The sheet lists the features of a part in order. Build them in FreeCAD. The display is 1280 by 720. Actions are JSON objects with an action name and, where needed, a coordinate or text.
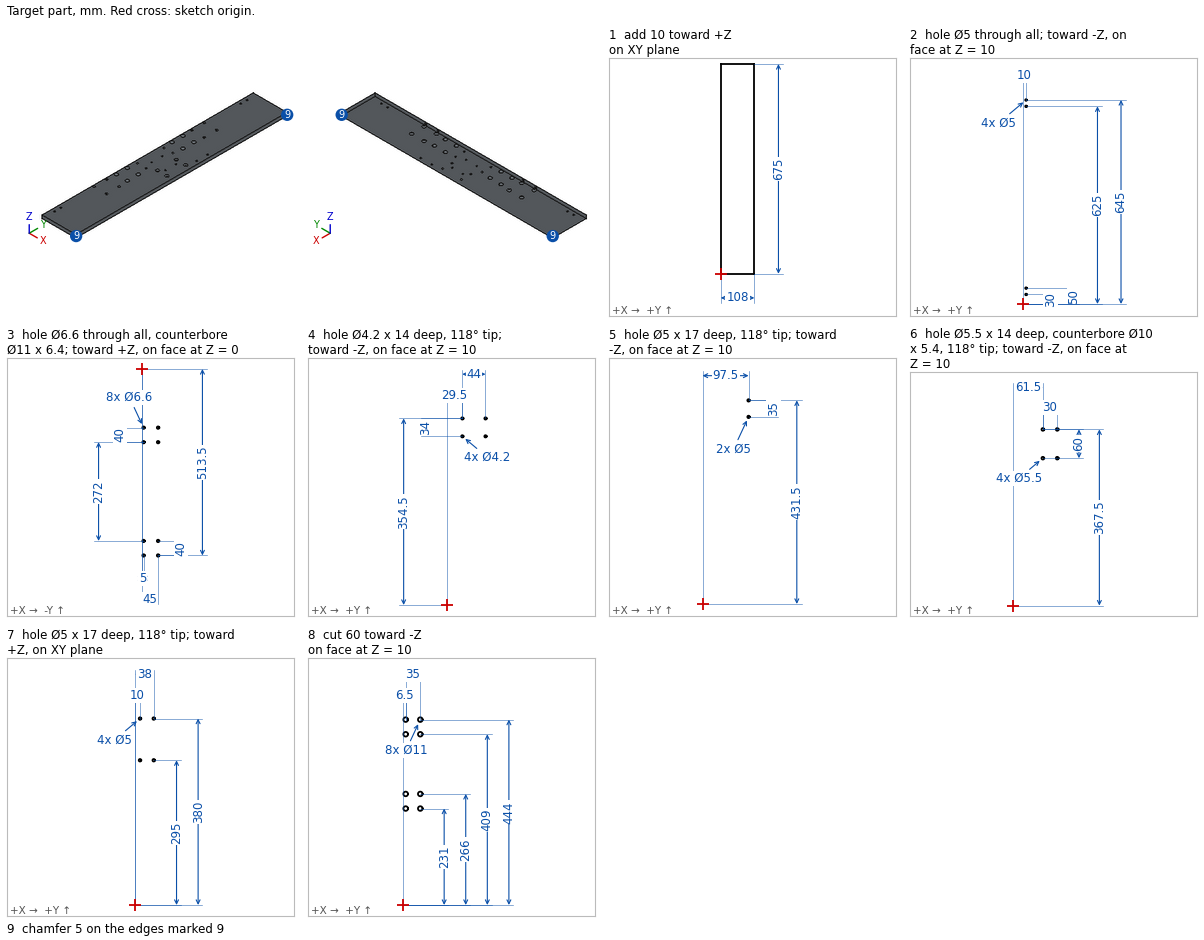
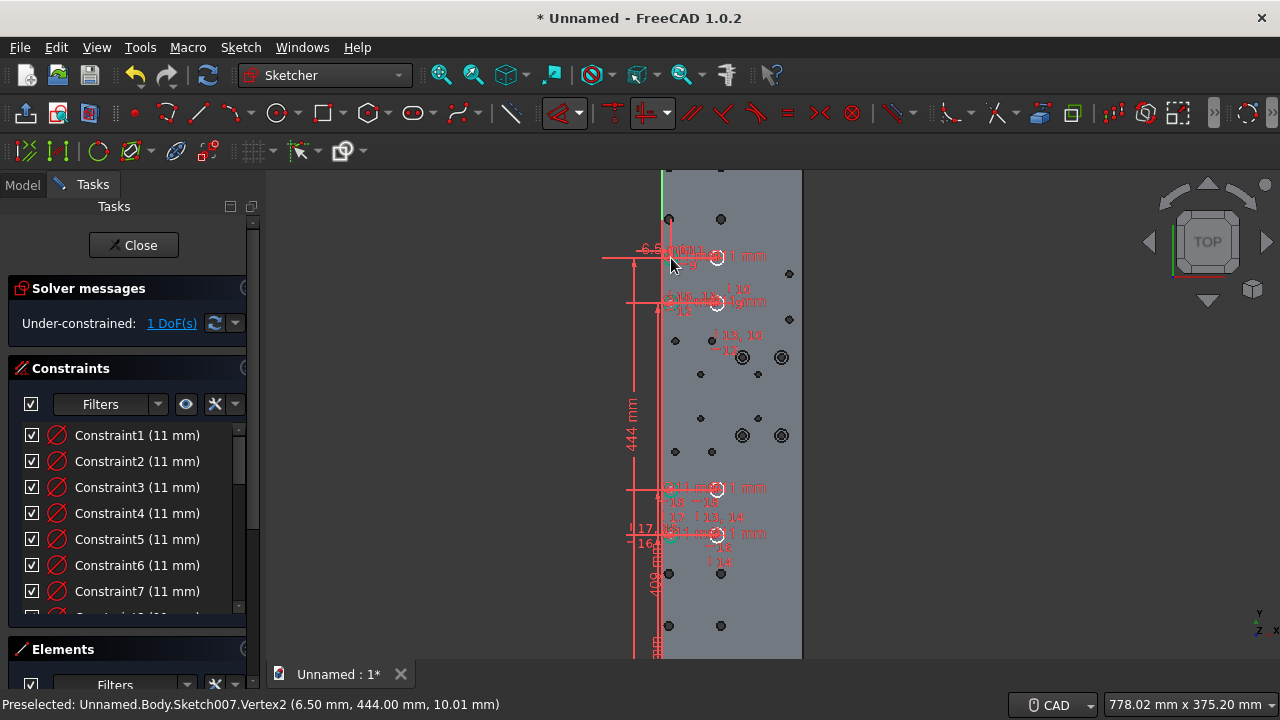
{"action": "key", "text": "l"}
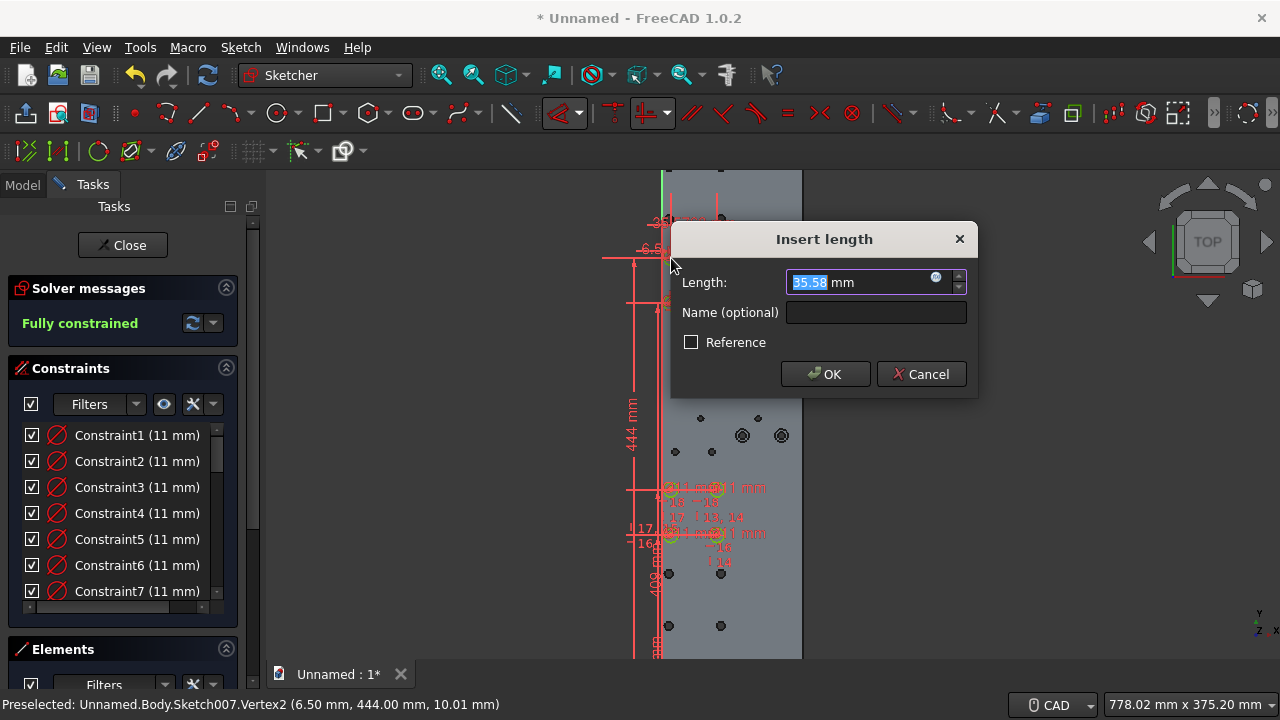
{"action": "type", "text": "35"}
{"action": "key", "text": "Return"}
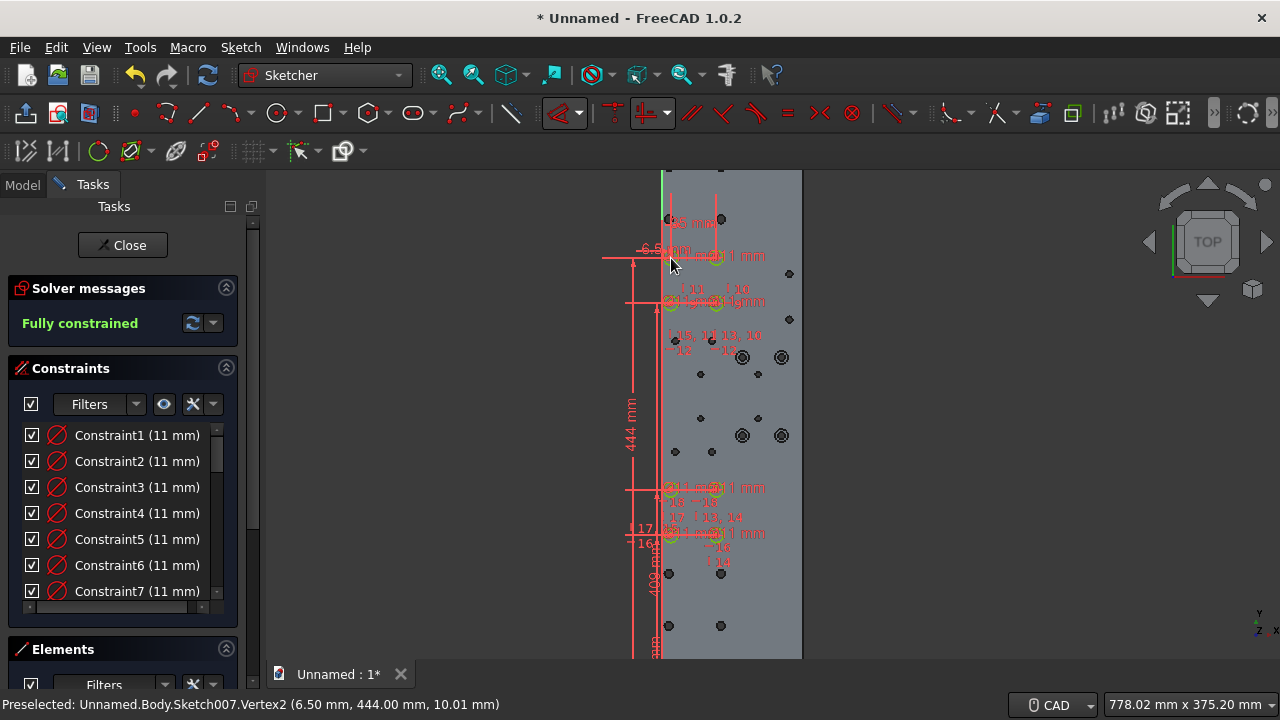
{"action": "left_click", "coordinate": [123, 245]}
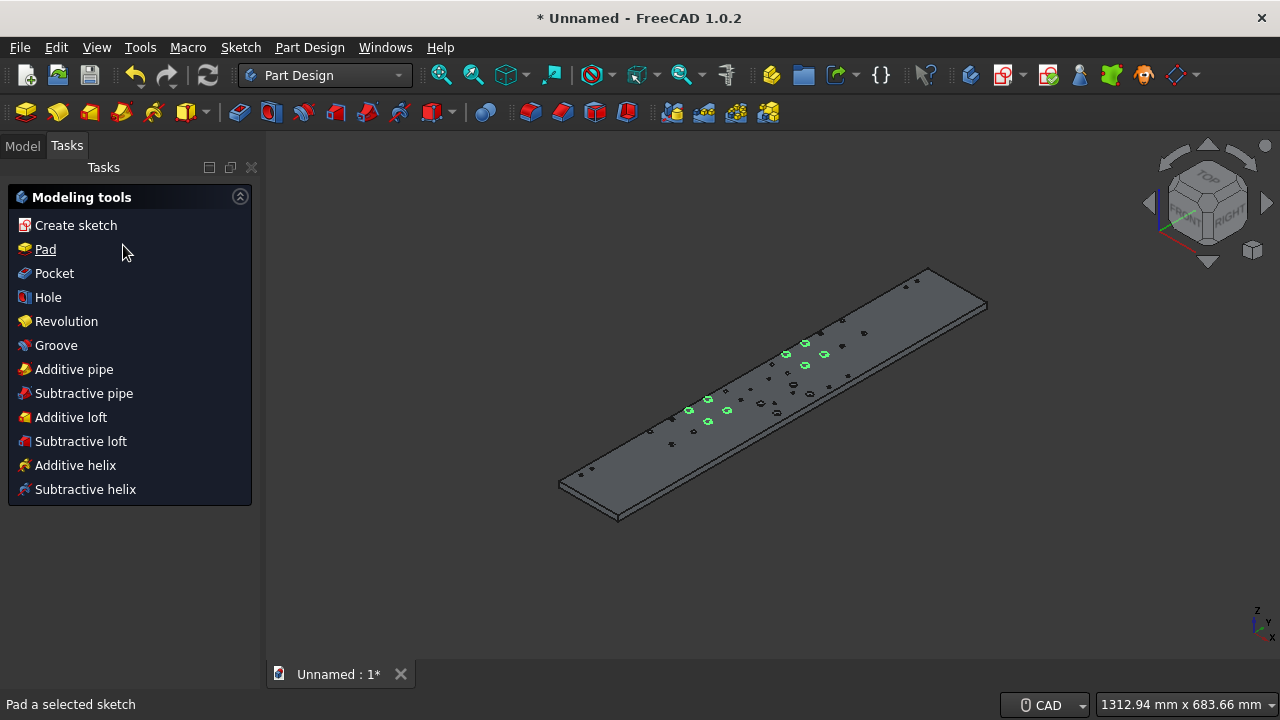
{"action": "left_click", "coordinate": [240, 112]}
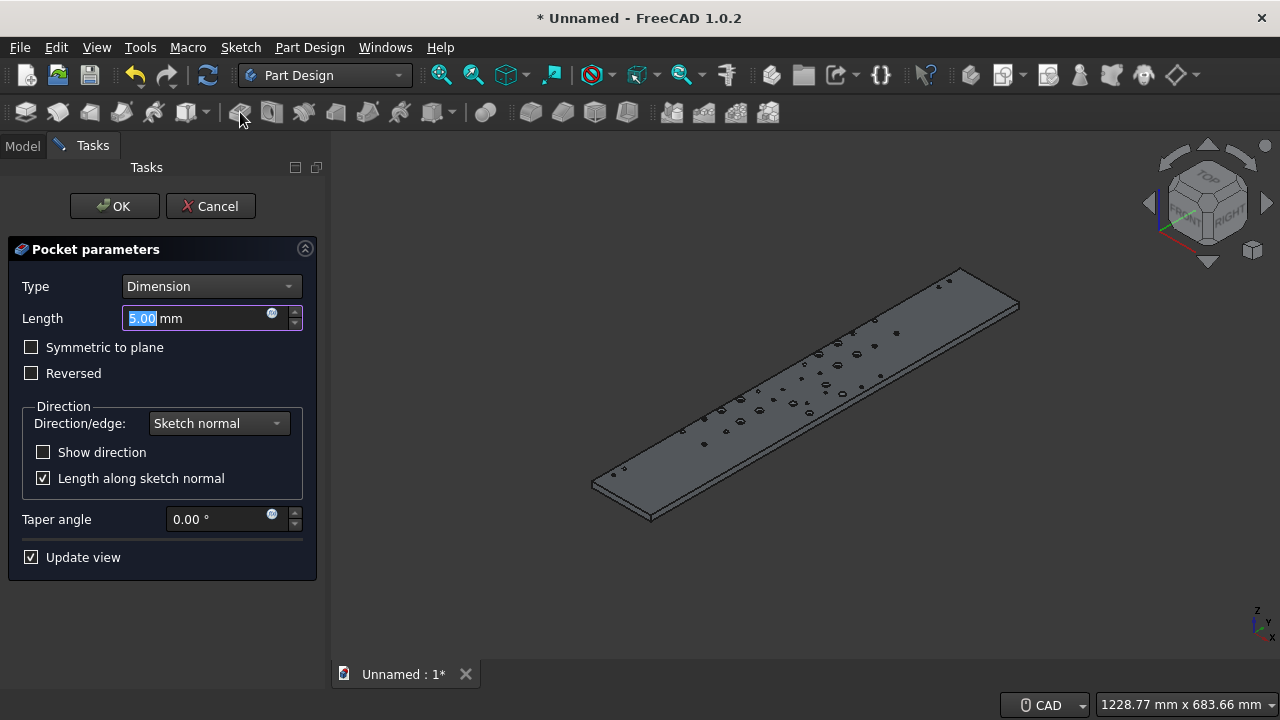
{"action": "type", "text": "60"}
{"action": "key", "text": "Tab"}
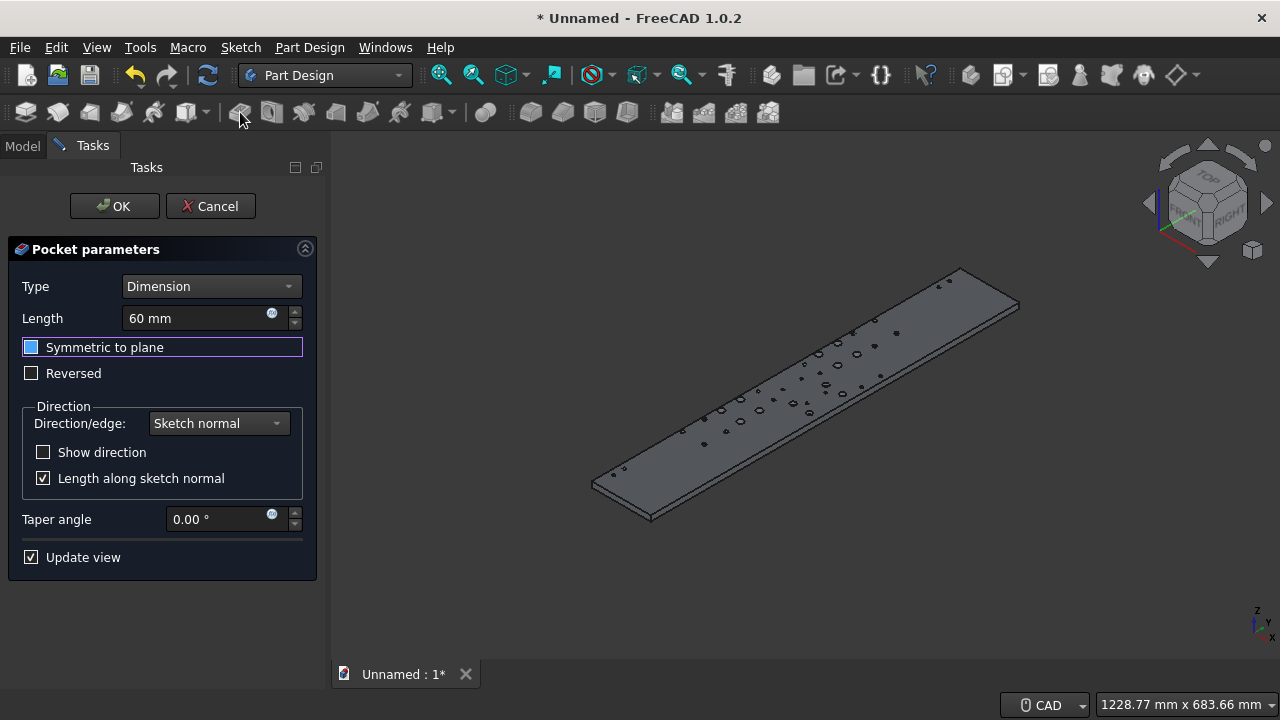
{"action": "left_click", "coordinate": [115, 206]}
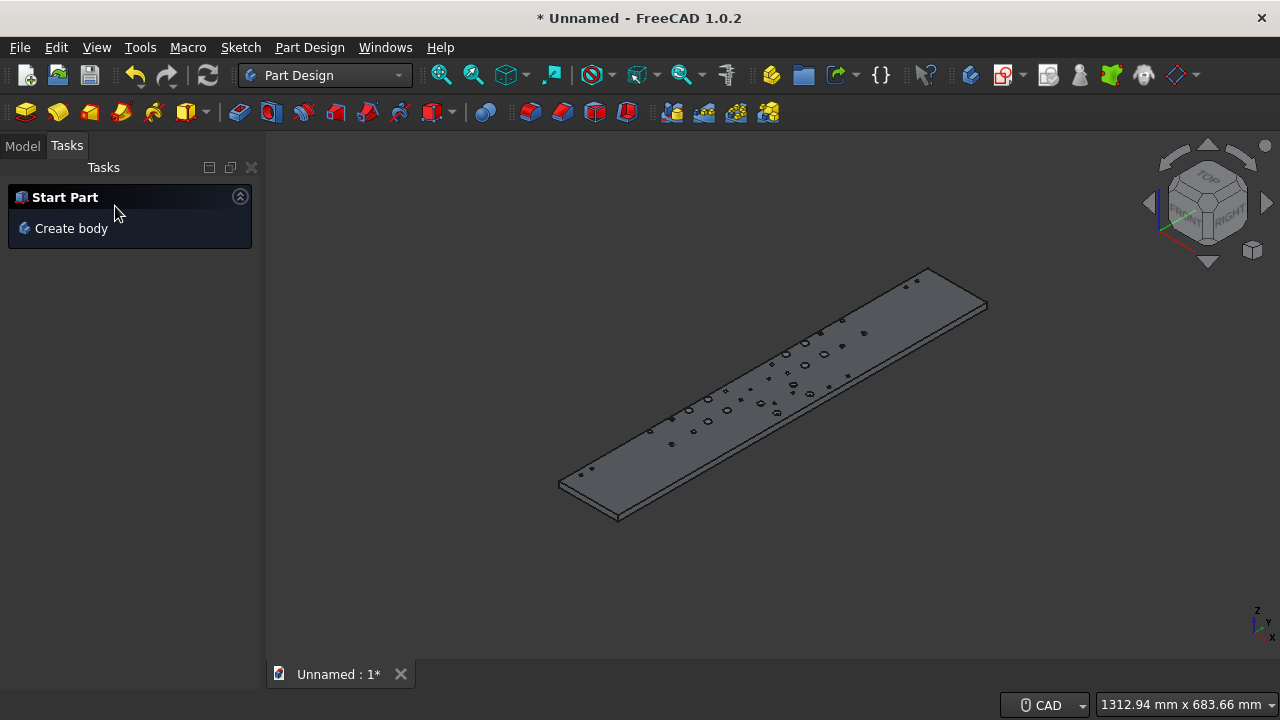
{"action": "scroll", "coordinate": [618, 517], "scroll_direction": "up", "scroll_amount": 9}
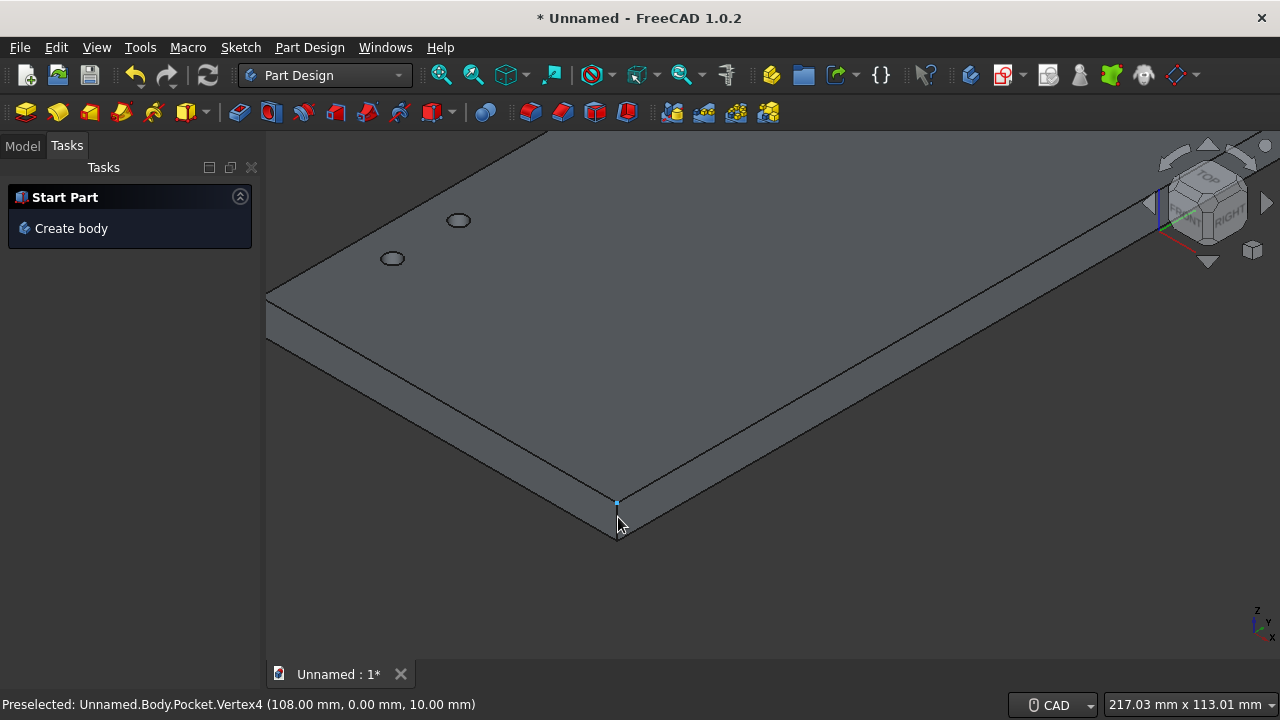
{"action": "left_click", "coordinate": [617, 521]}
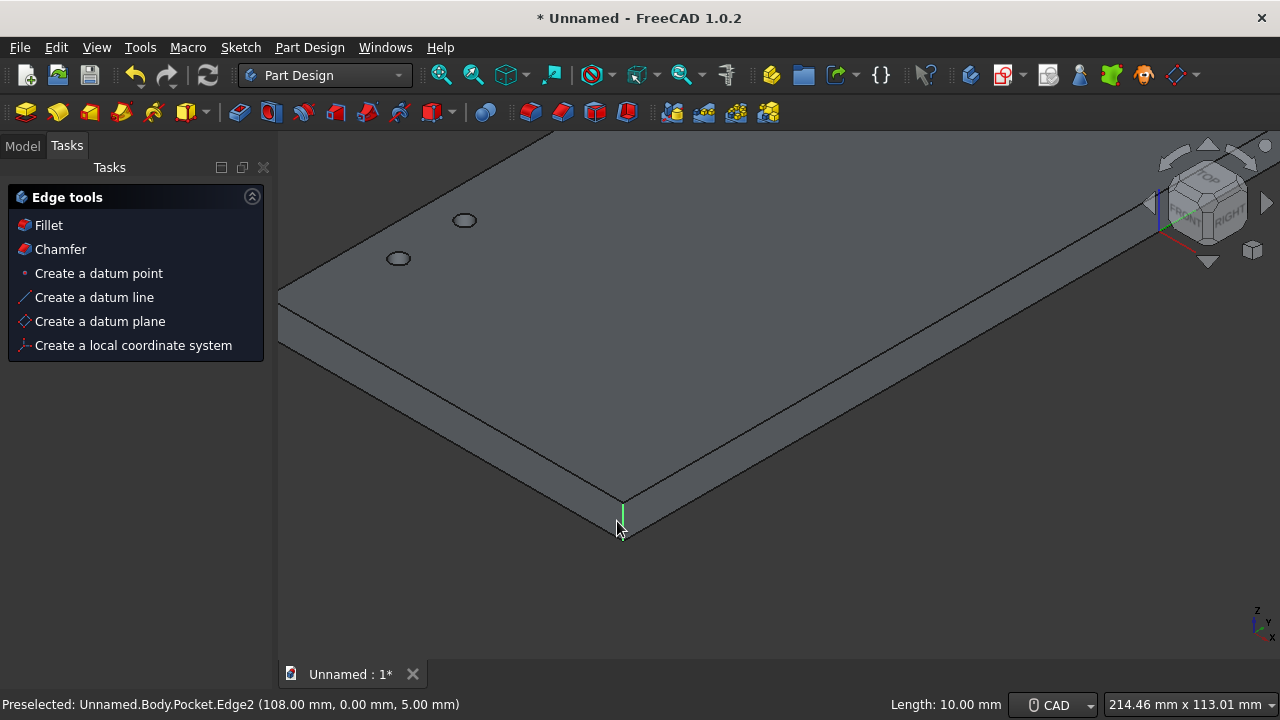
{"action": "left_click", "coordinate": [442, 76]}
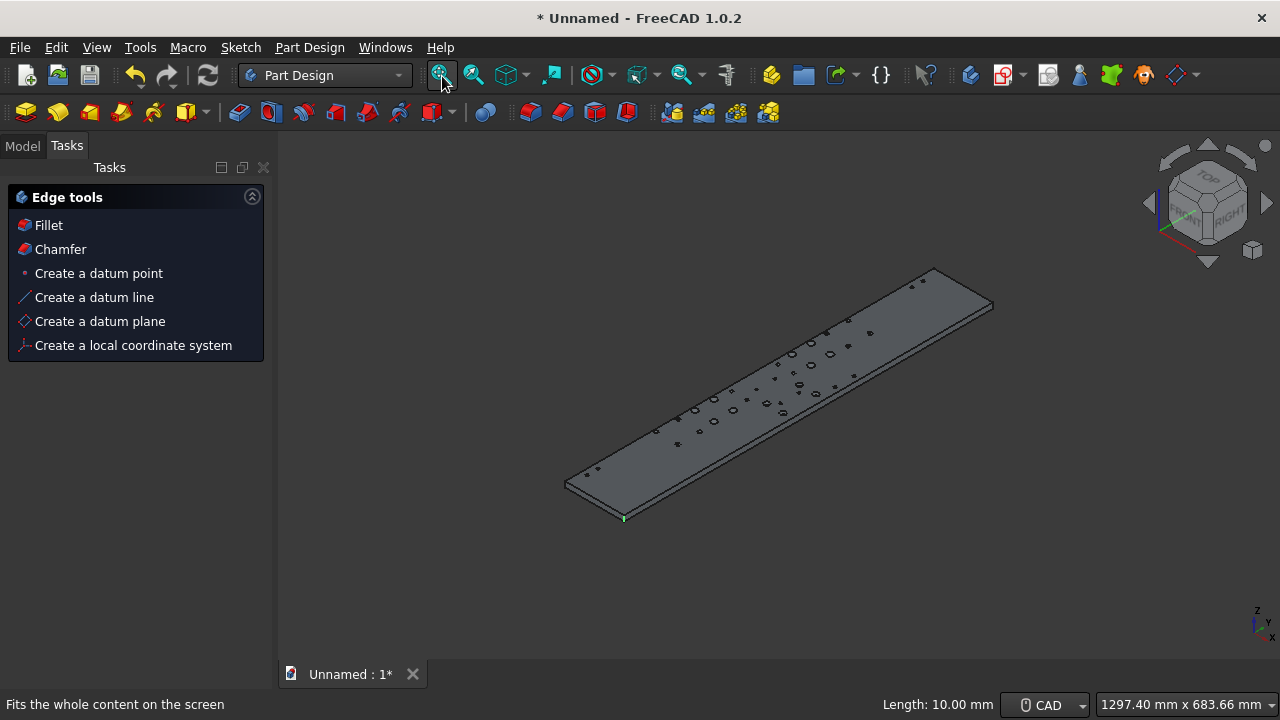
{"action": "key", "text": "2"}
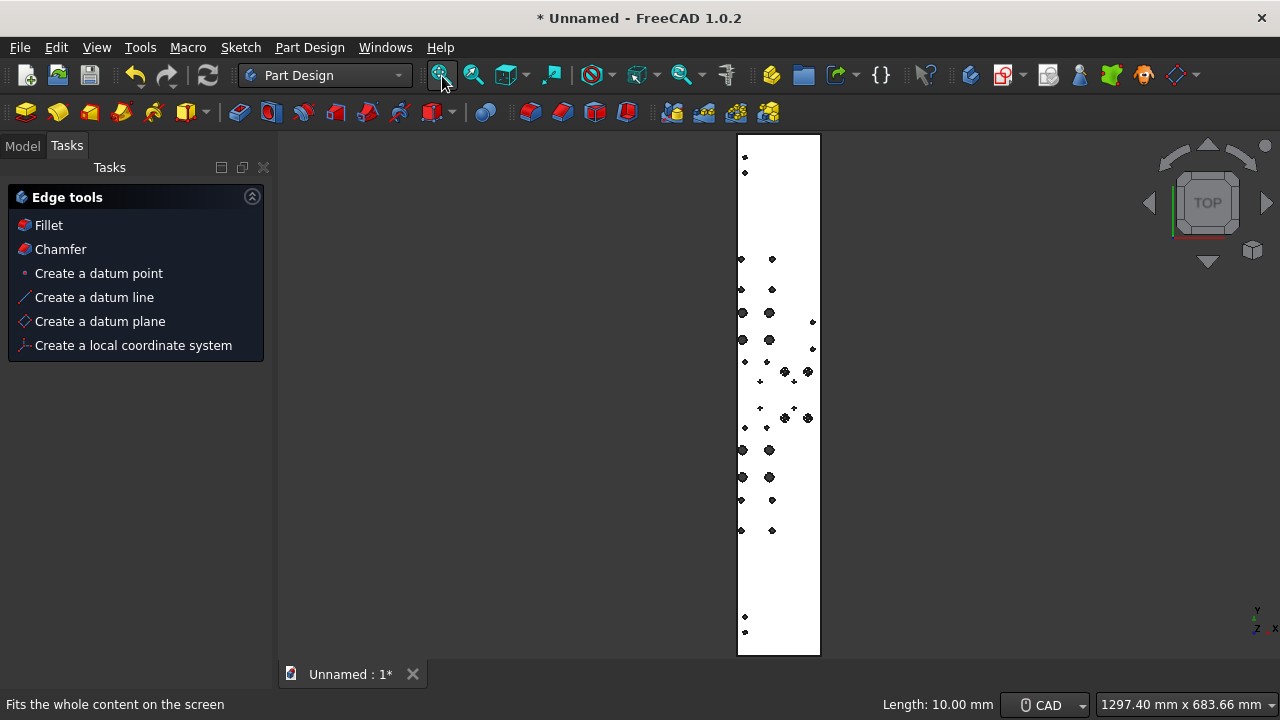
{"action": "key", "text": "0"}